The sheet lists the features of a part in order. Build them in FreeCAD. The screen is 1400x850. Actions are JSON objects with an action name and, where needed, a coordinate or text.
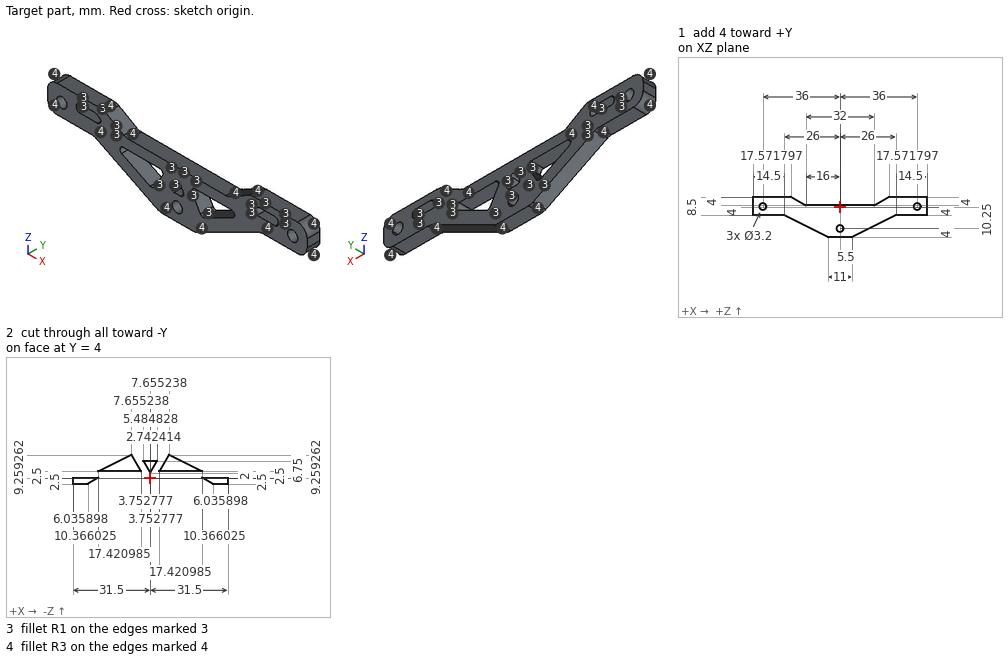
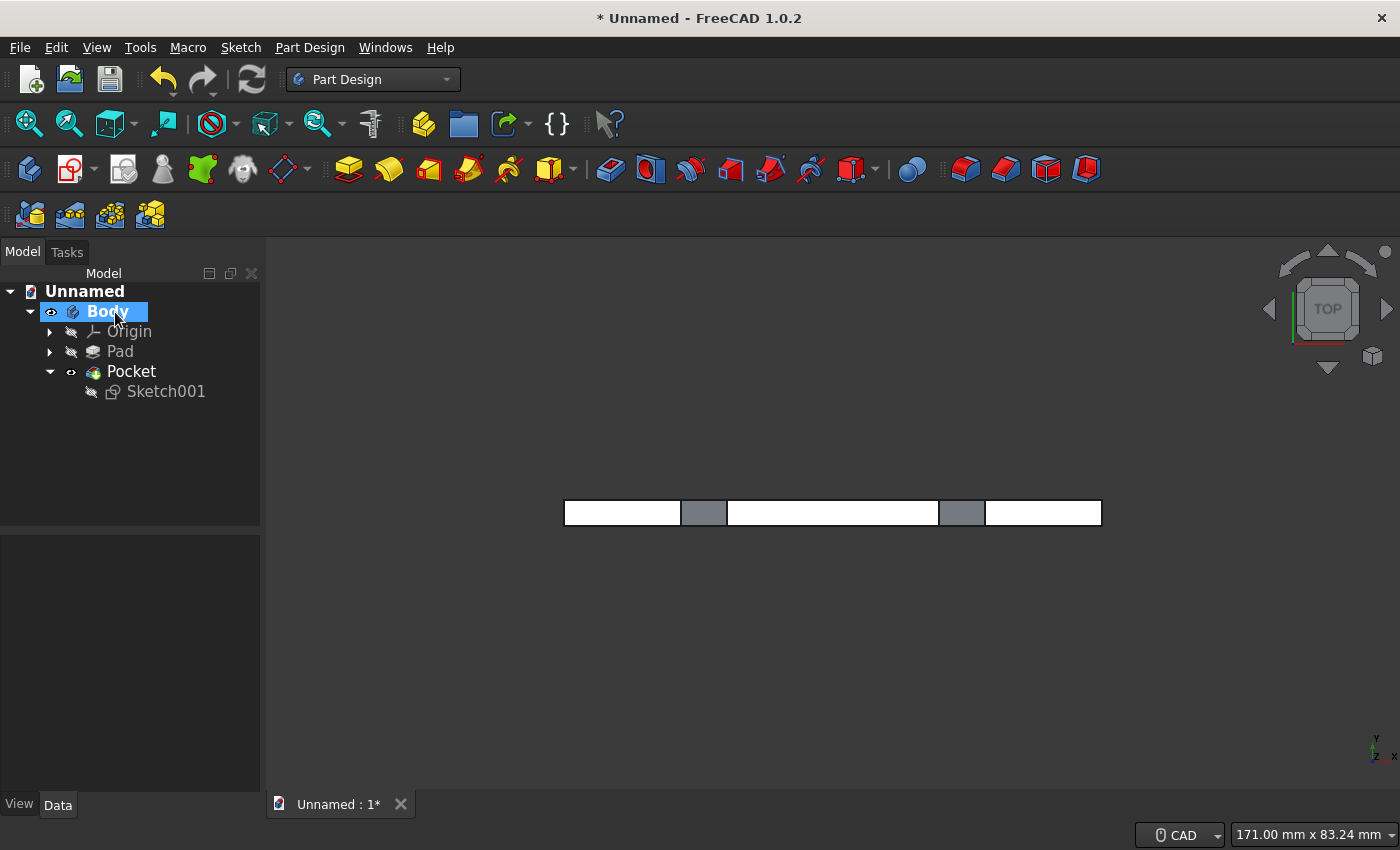
{"action": "key", "text": "1"}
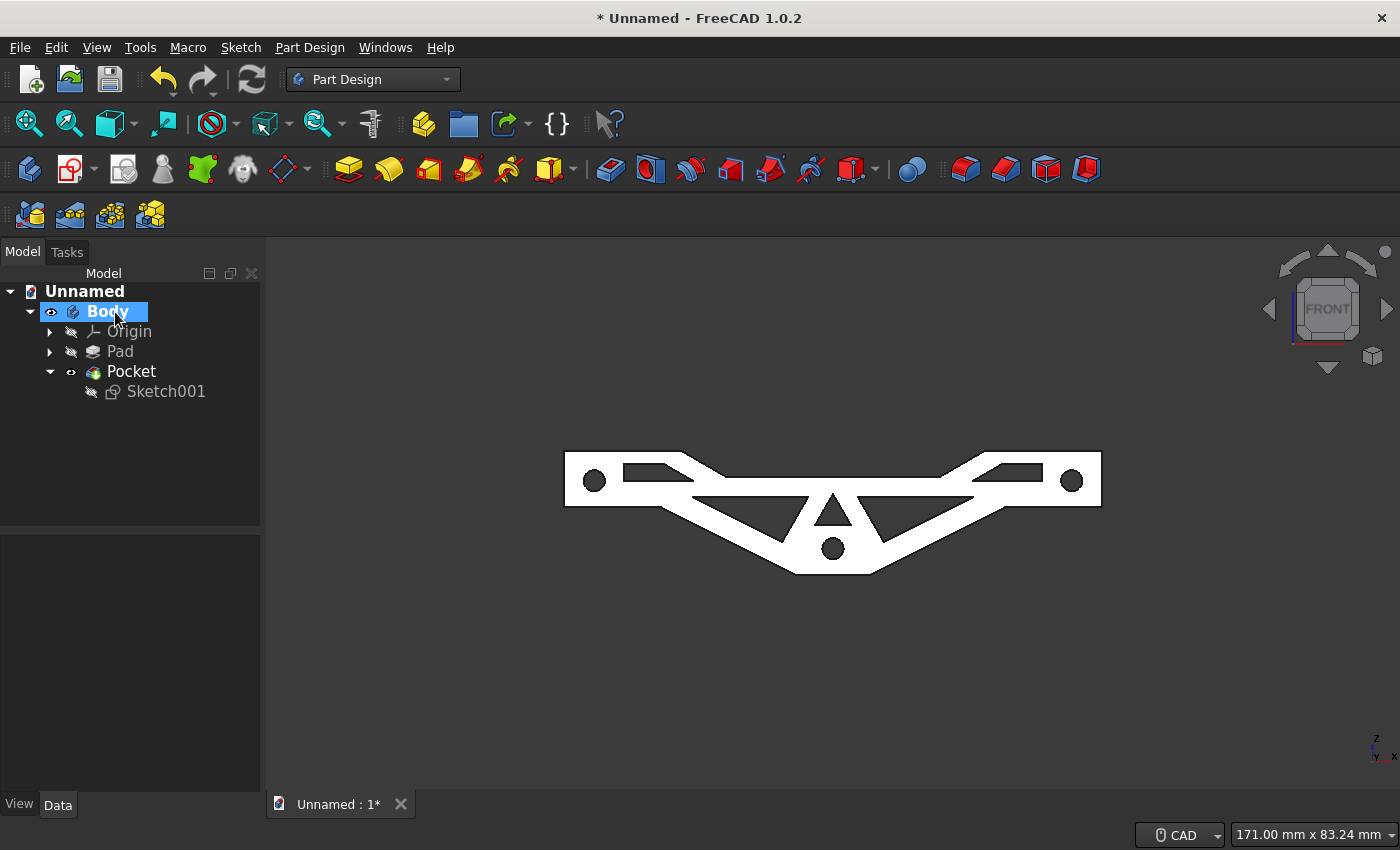
{"action": "key", "text": "3"}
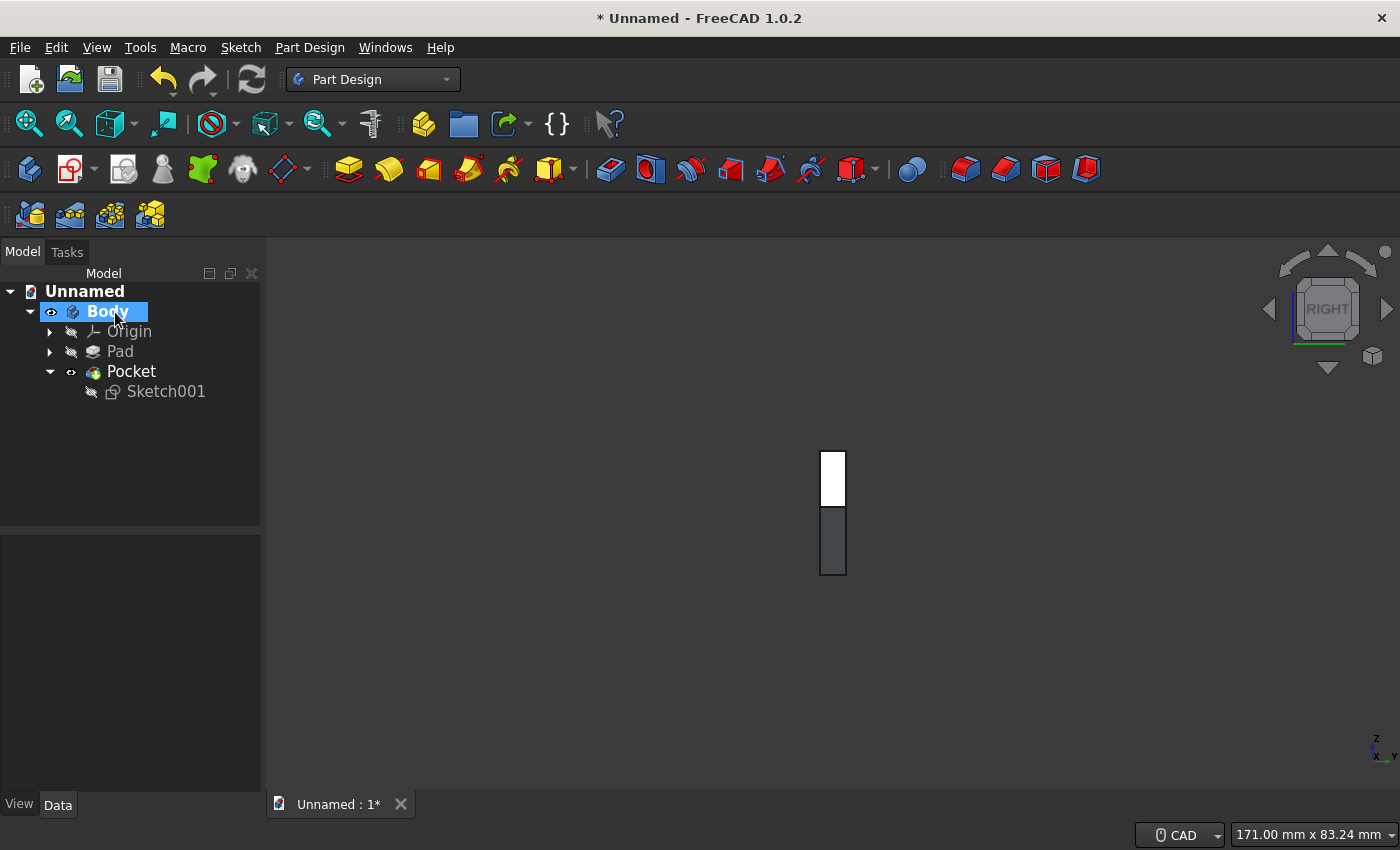
{"action": "left_click", "coordinate": [30, 124]}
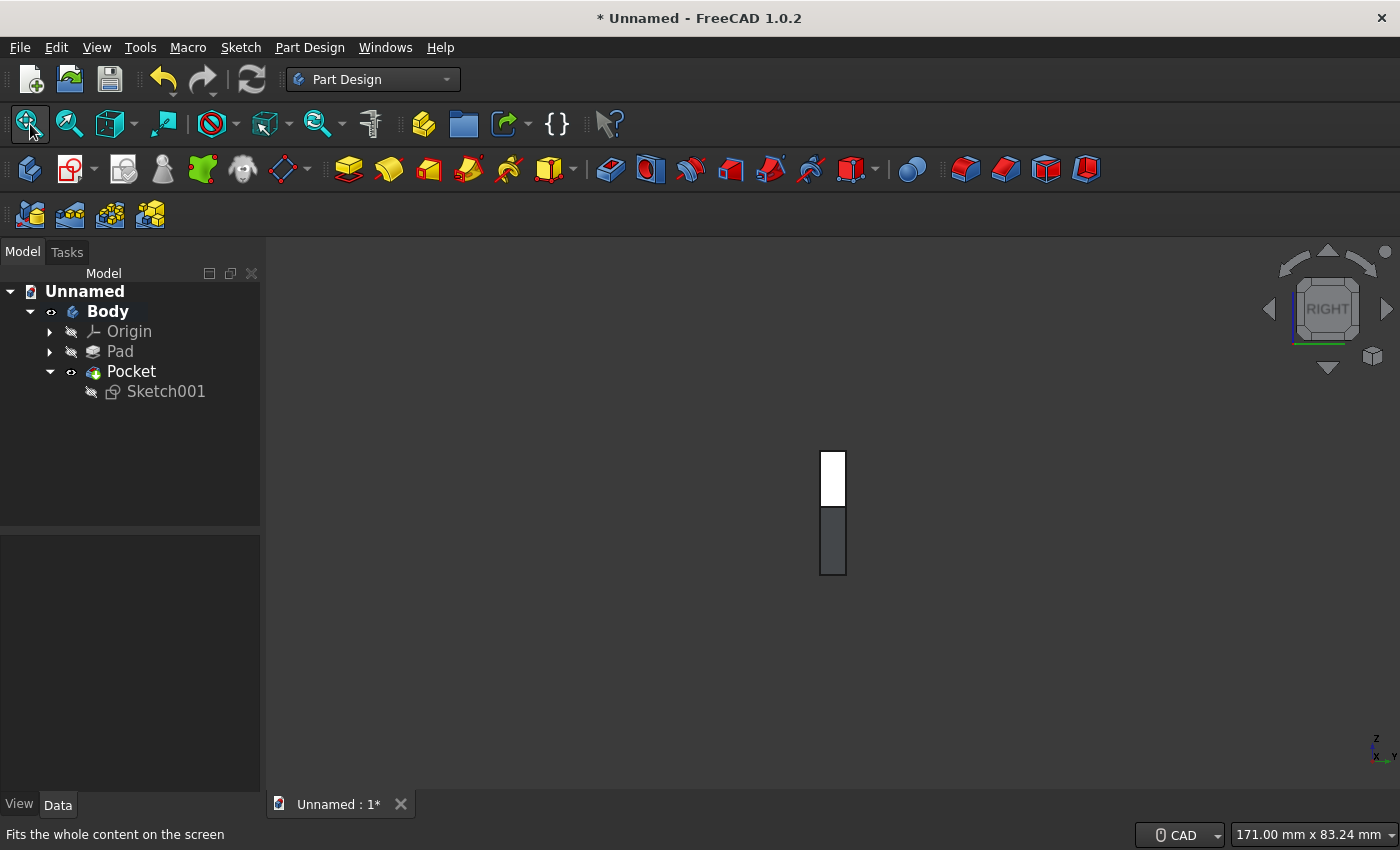
{"action": "key", "text": "5"}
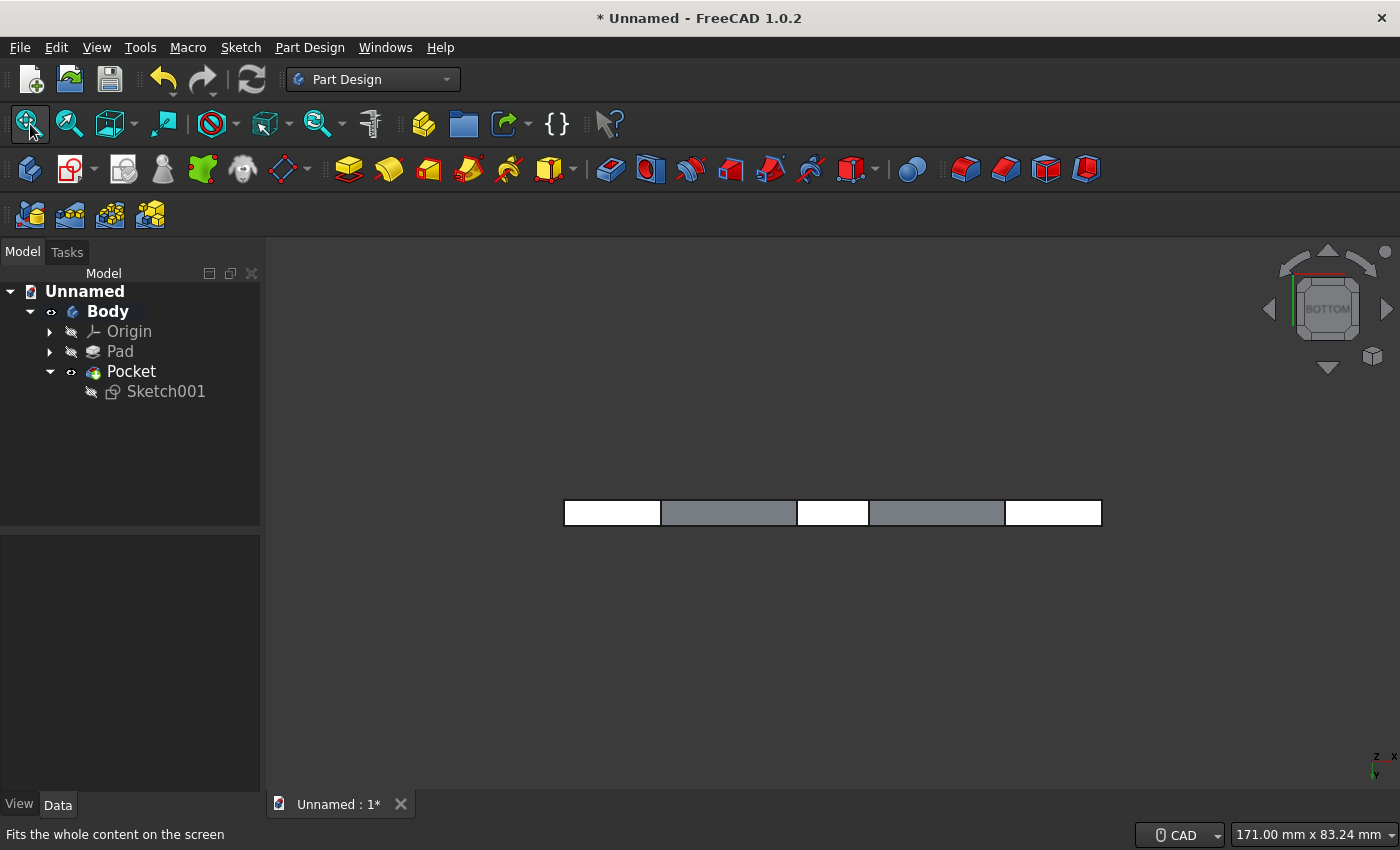
{"action": "key", "text": "4"}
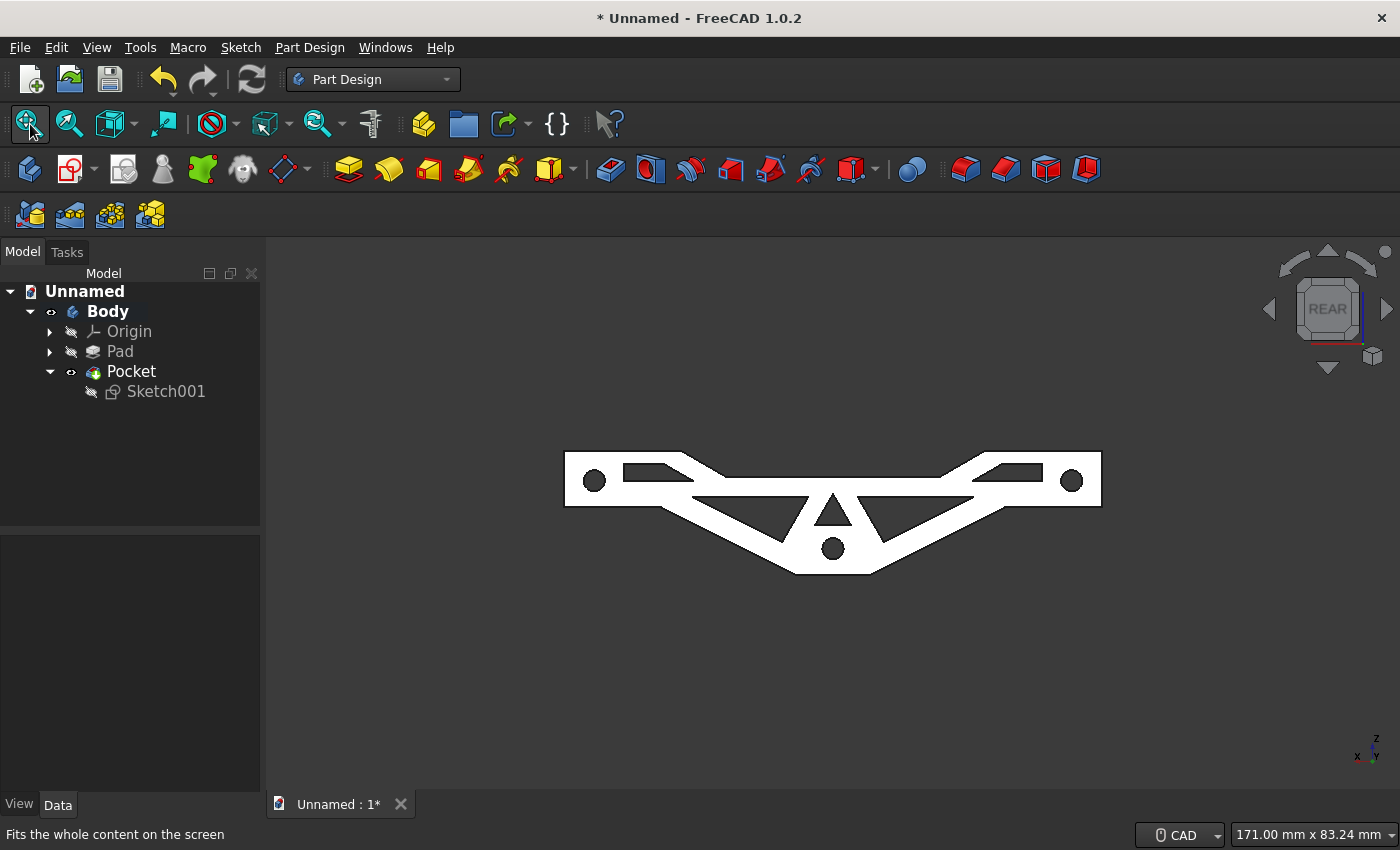
{"action": "key", "text": "6"}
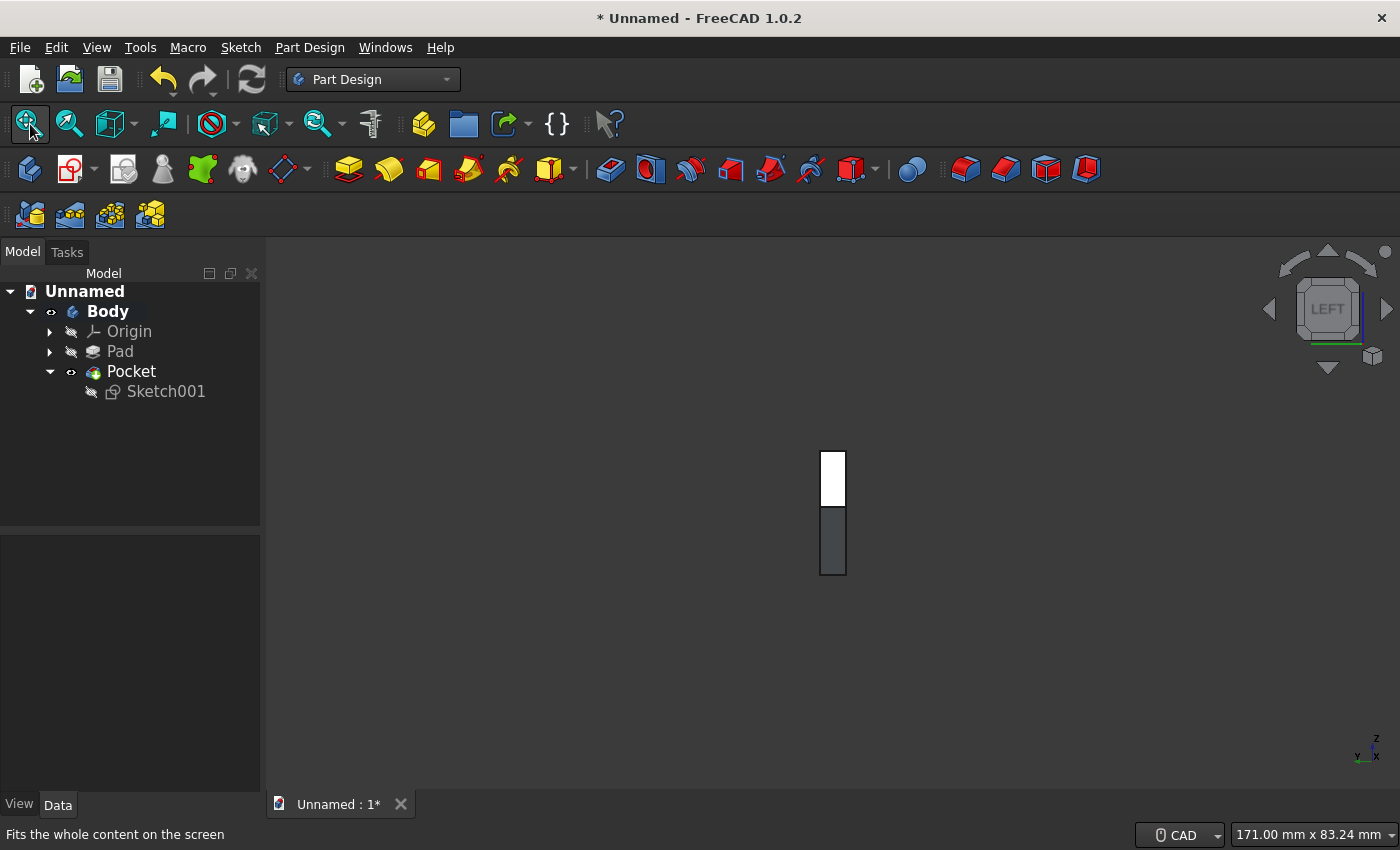
{"action": "left_click", "coordinate": [30, 124]}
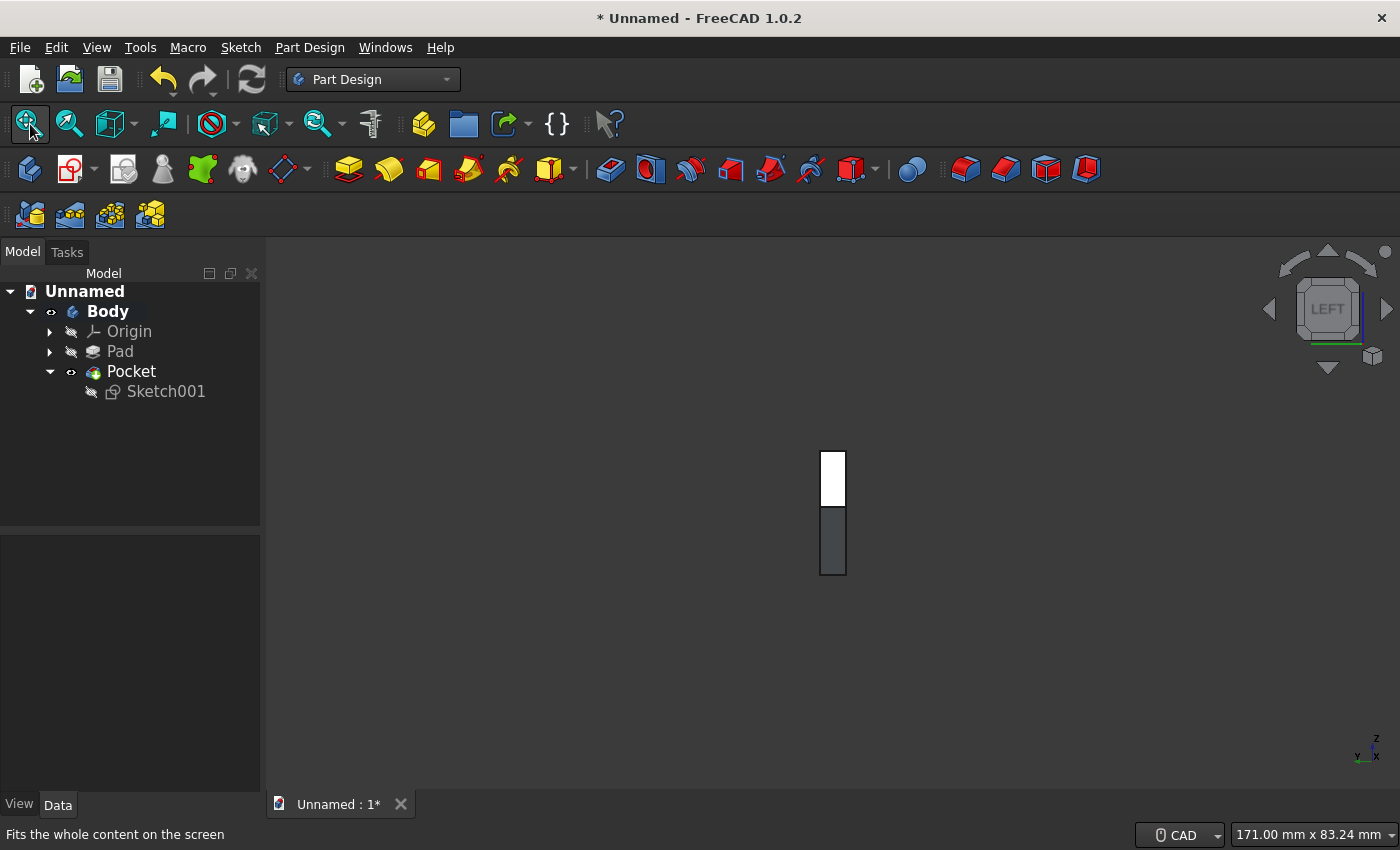
{"action": "key", "text": "v 3"}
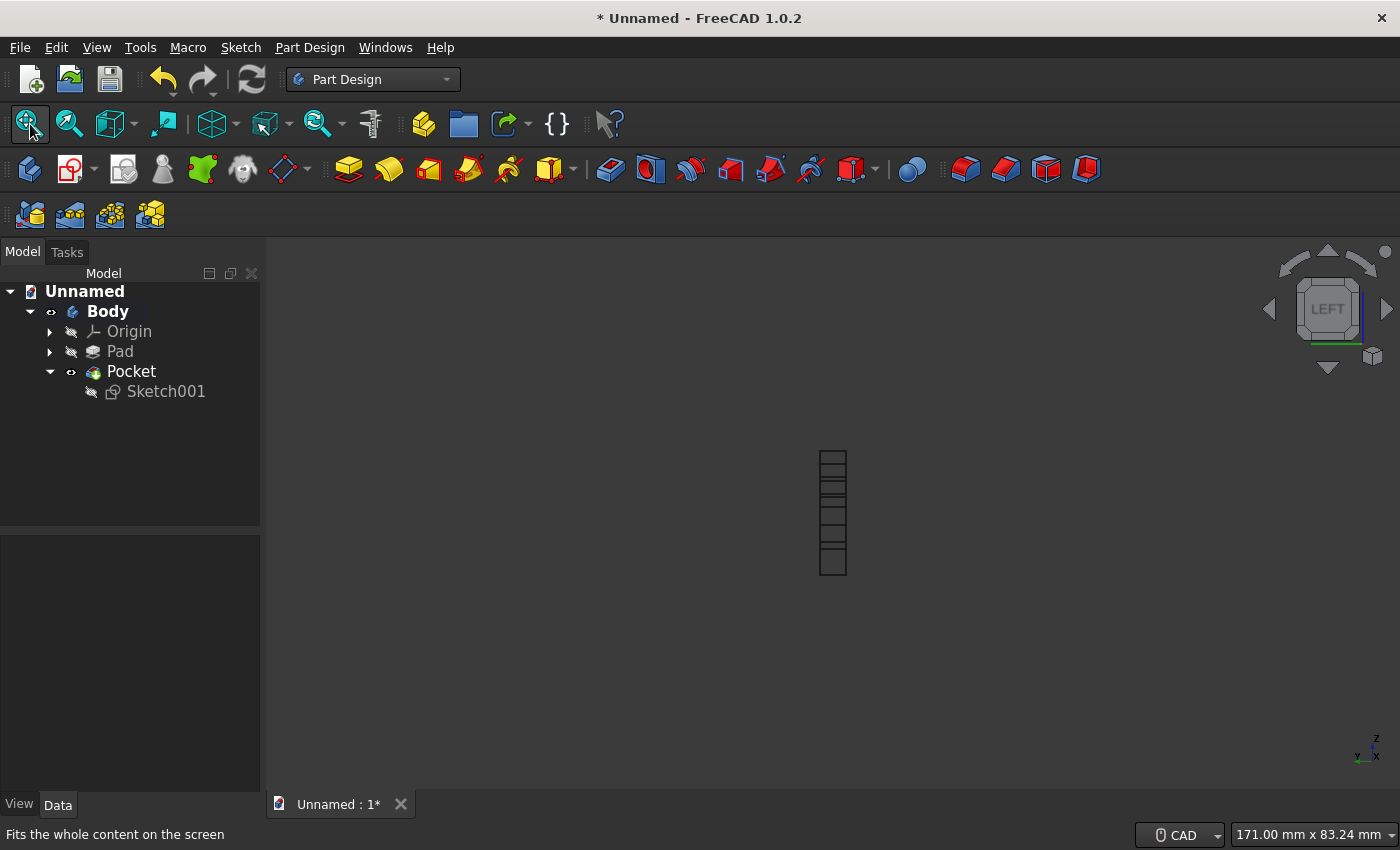
{"action": "key", "text": "0"}